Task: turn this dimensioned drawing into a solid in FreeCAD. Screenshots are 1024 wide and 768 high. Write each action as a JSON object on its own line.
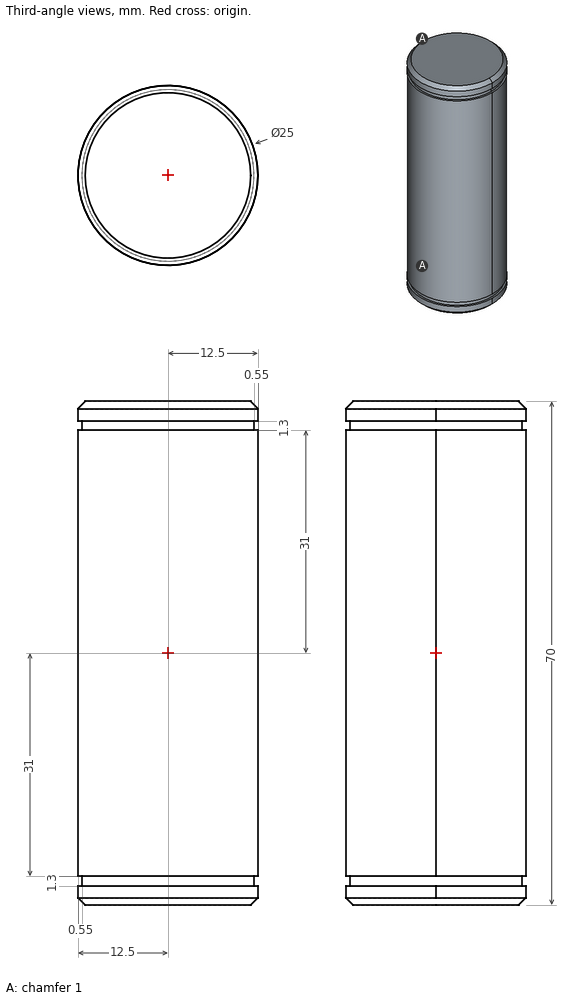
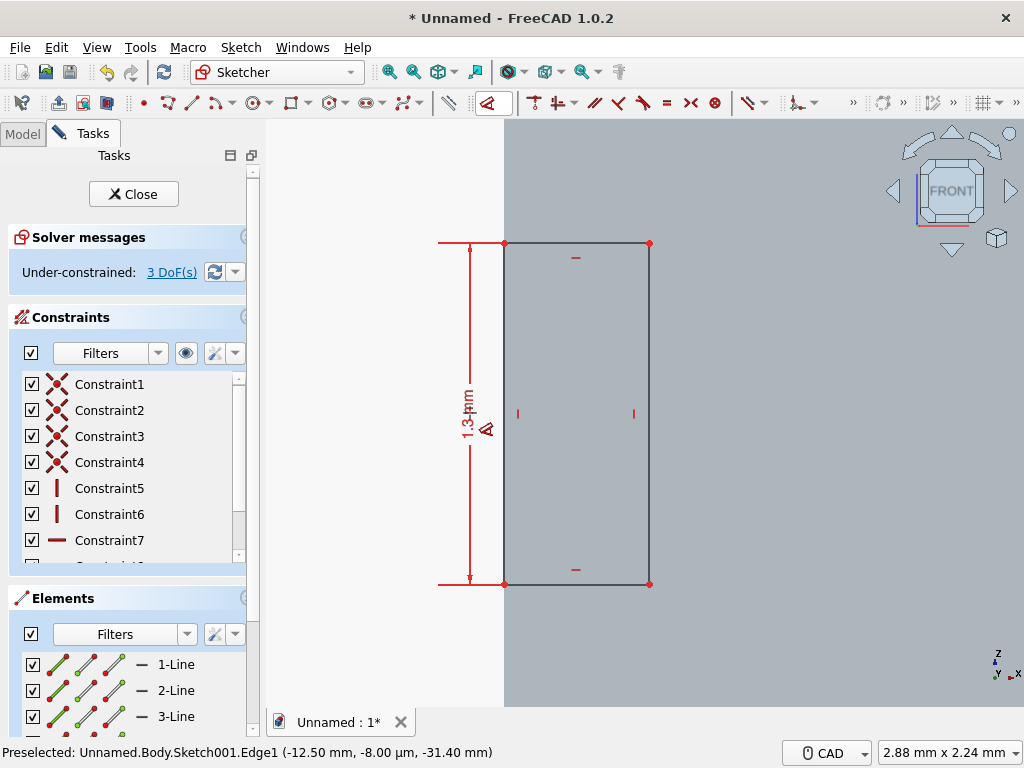
{"action": "left_click", "coordinate": [504, 243]}
{"action": "left_click", "coordinate": [470, 195]}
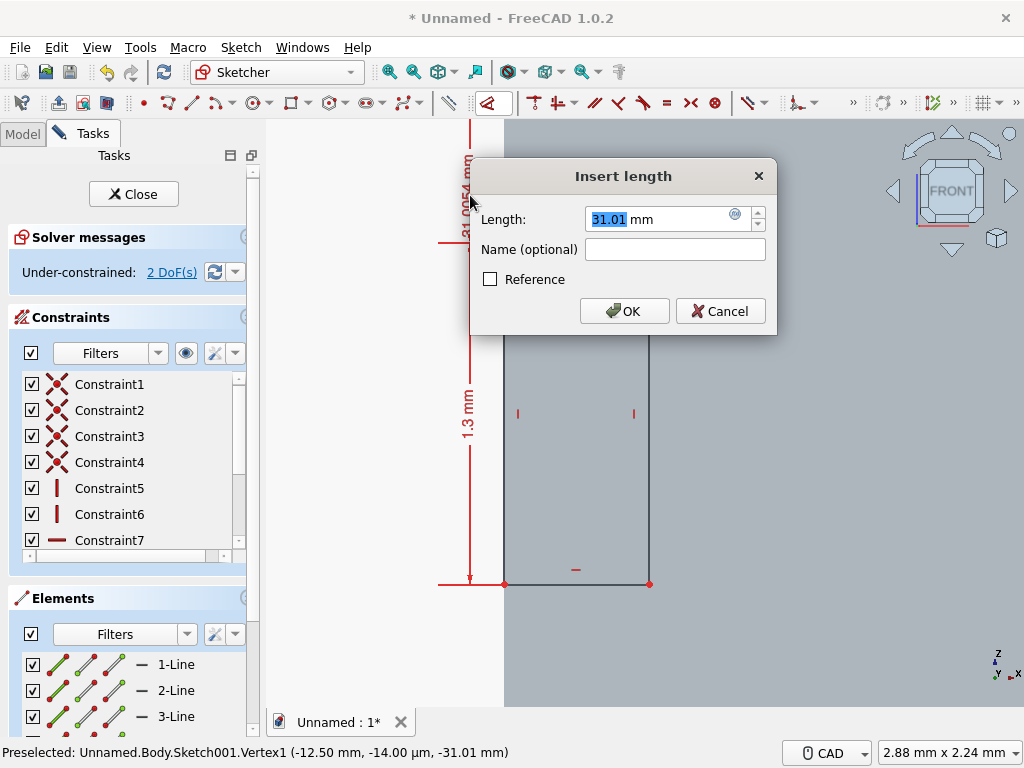
{"action": "type", "text": "31"}
{"action": "key", "text": "Return"}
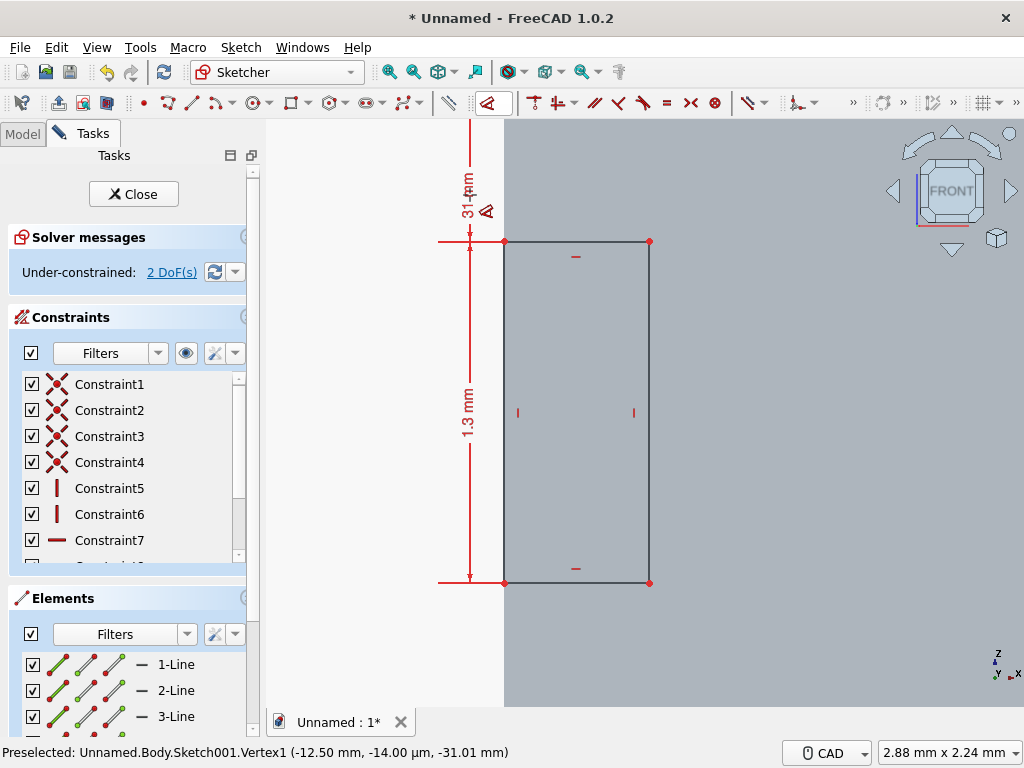
{"action": "left_click", "coordinate": [548, 583]}
{"action": "left_click", "coordinate": [577, 617]}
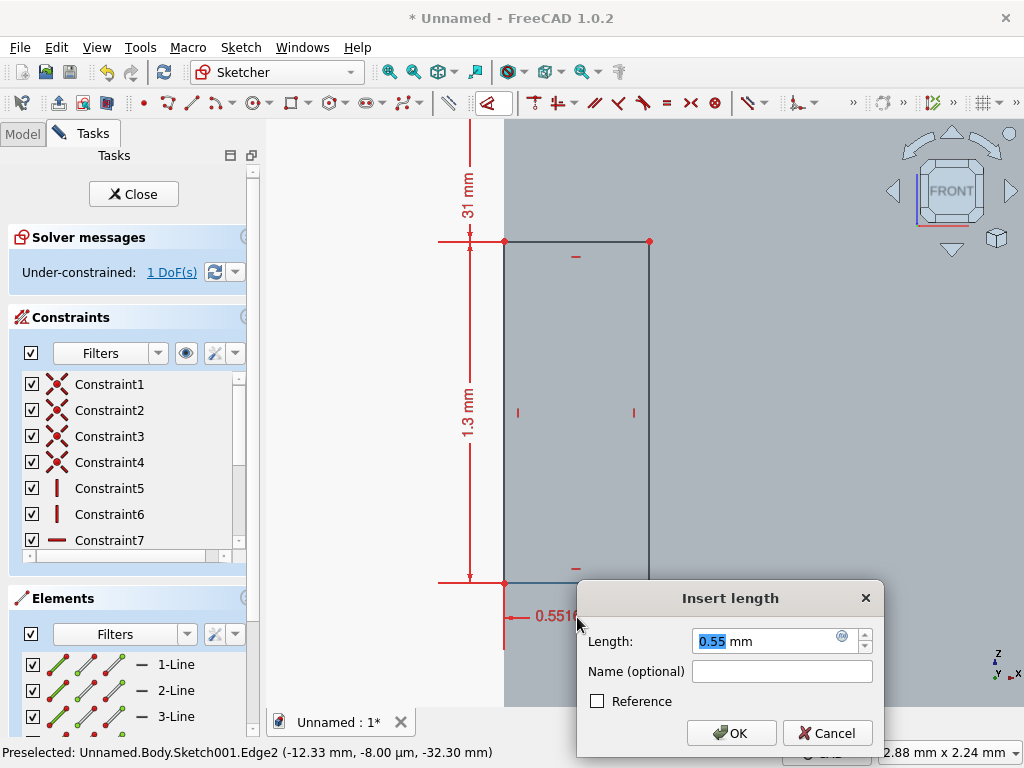
{"action": "type", "text": "0.55"}
{"action": "key", "text": "Return"}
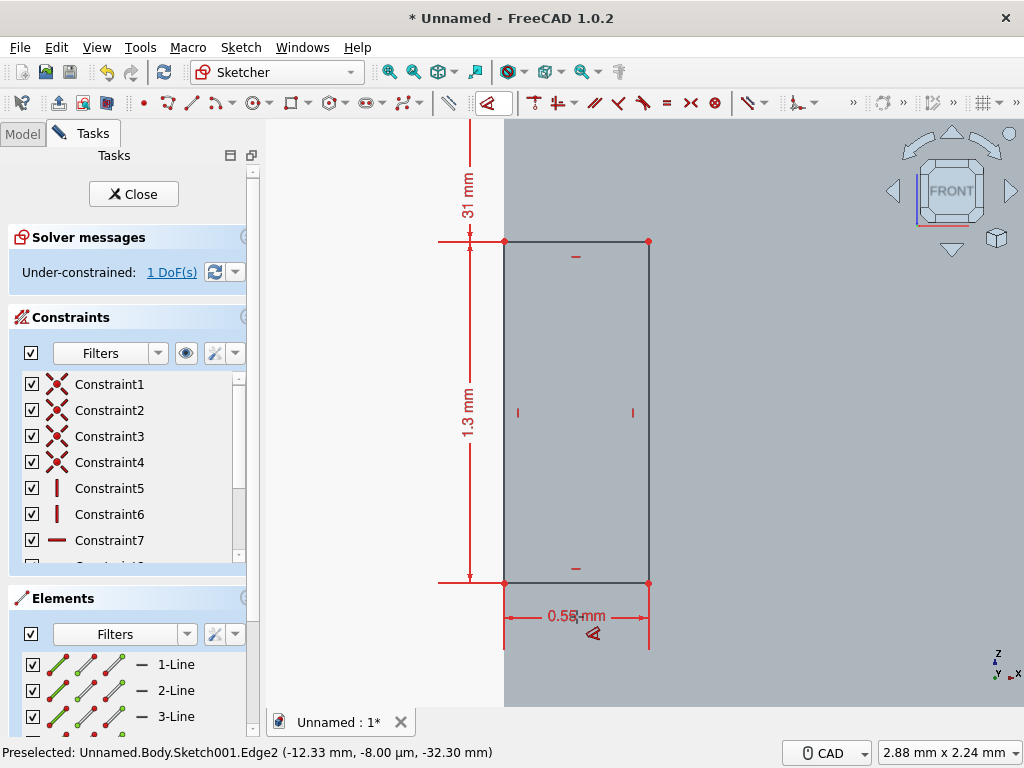
{"action": "left_click", "coordinate": [504, 242]}
{"action": "left_click", "coordinate": [682, 276]}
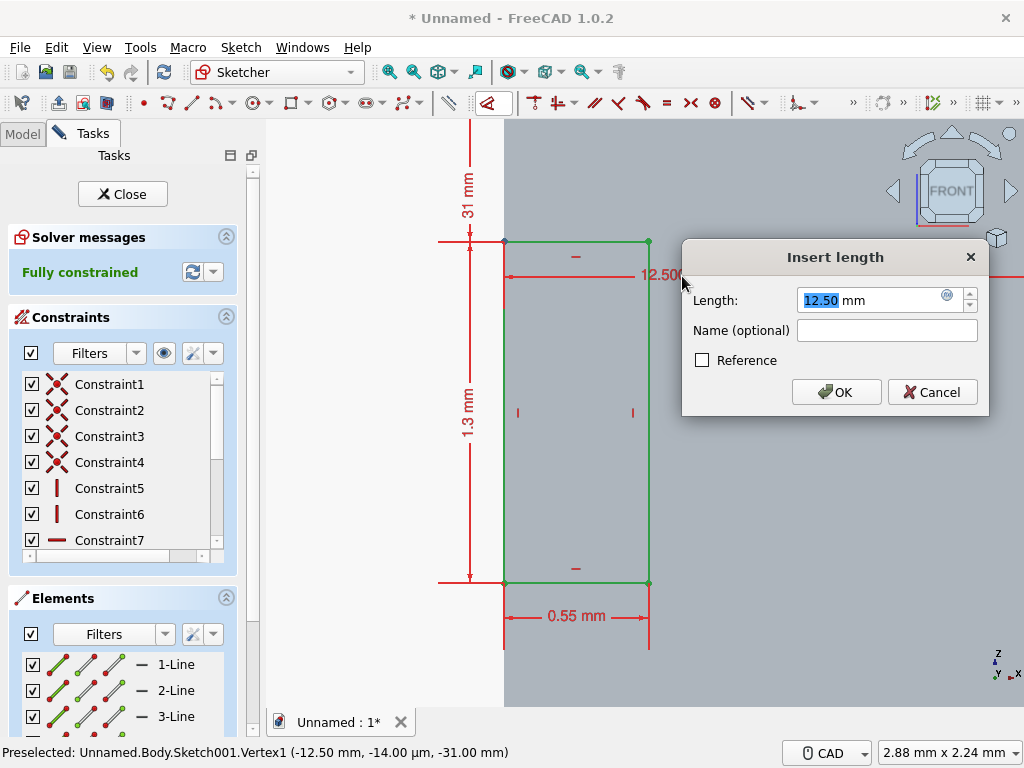
{"action": "type", "text": "12.5"}
{"action": "key", "text": "Return"}
{"action": "key", "text": "Escape"}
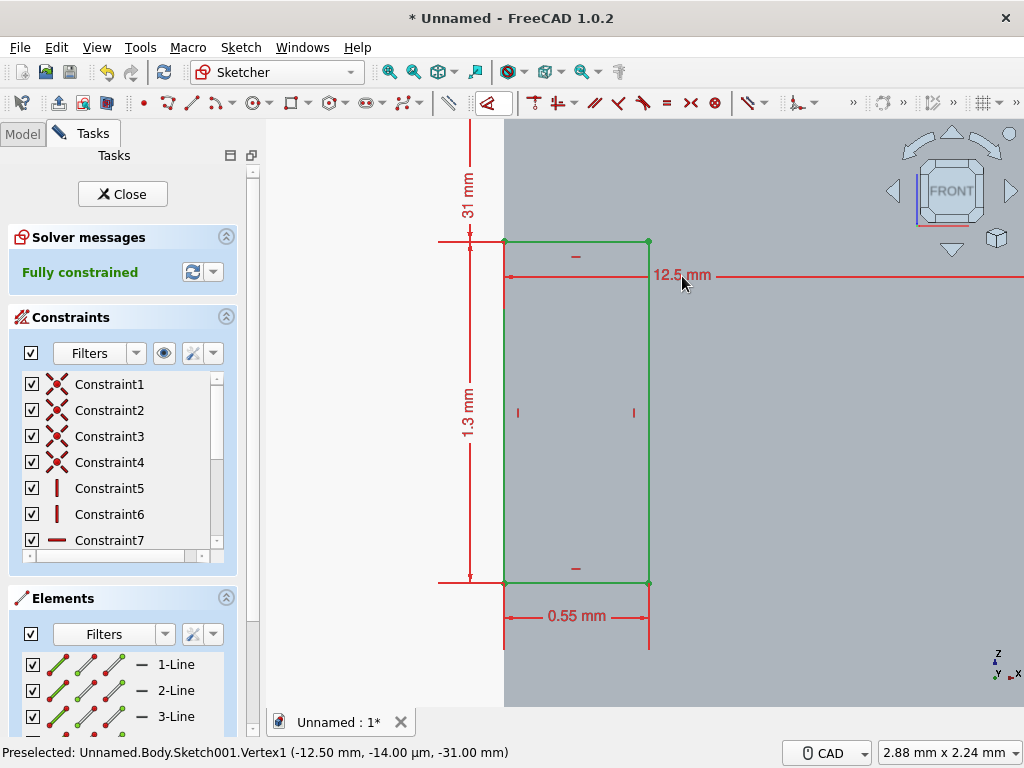
{"action": "left_click", "coordinate": [123, 194]}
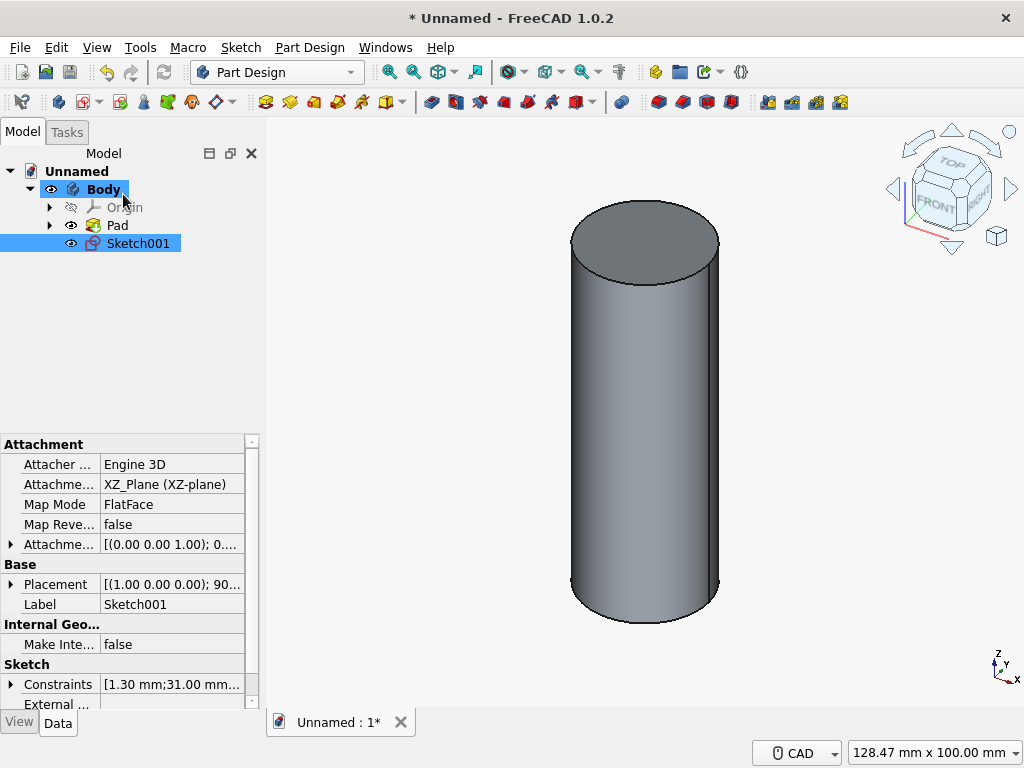
{"action": "left_click", "coordinate": [480, 102]}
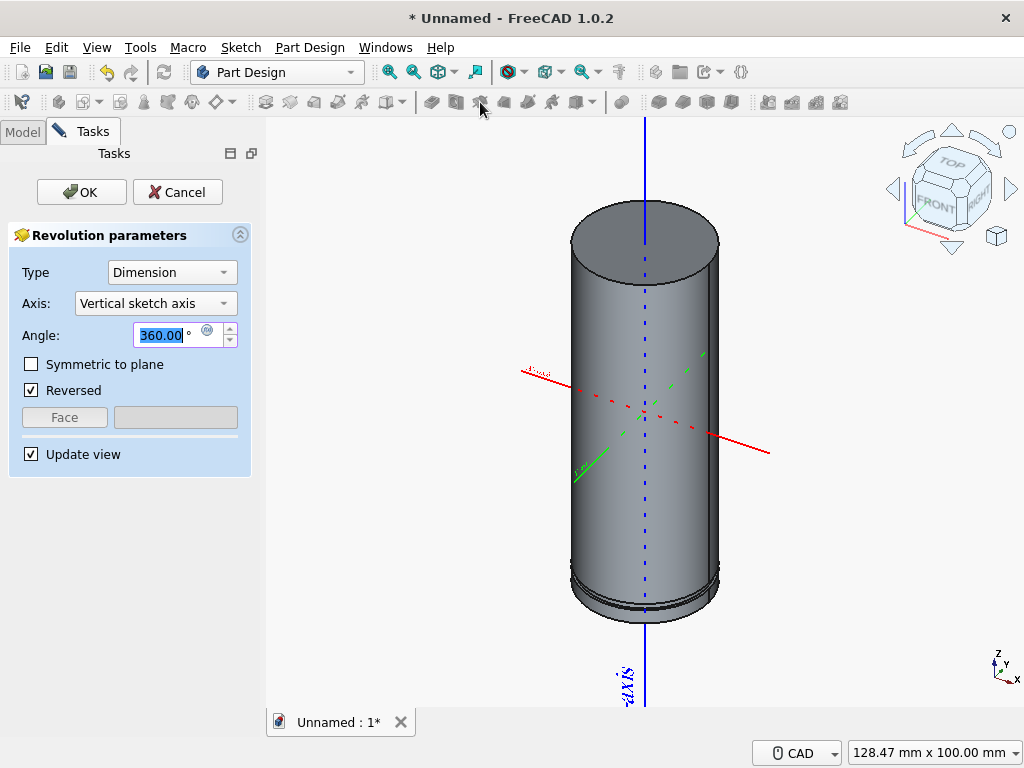
{"action": "left_click", "coordinate": [82, 192]}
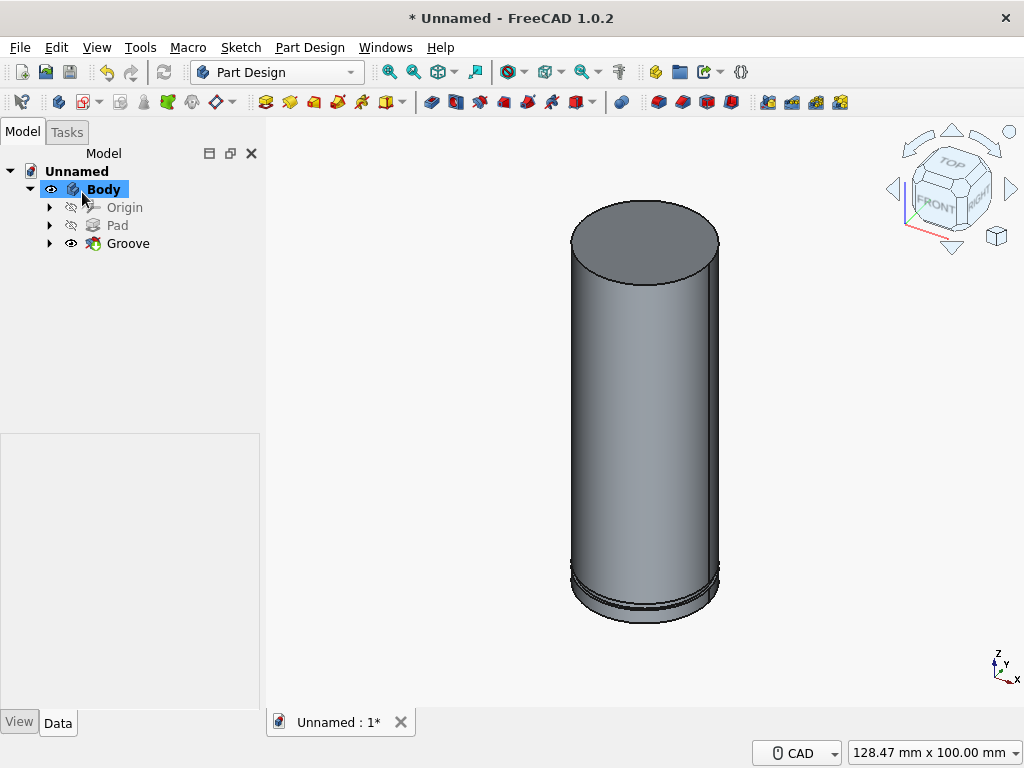
{"action": "left_click", "coordinate": [84, 102]}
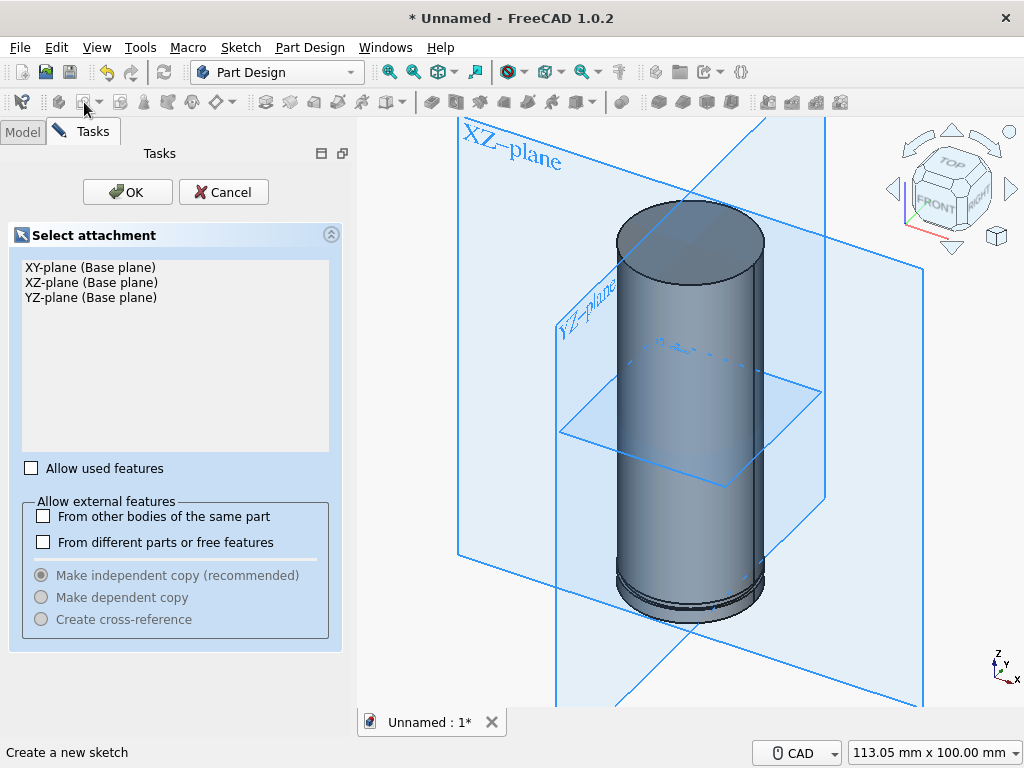
{"action": "left_click", "coordinate": [82, 282]}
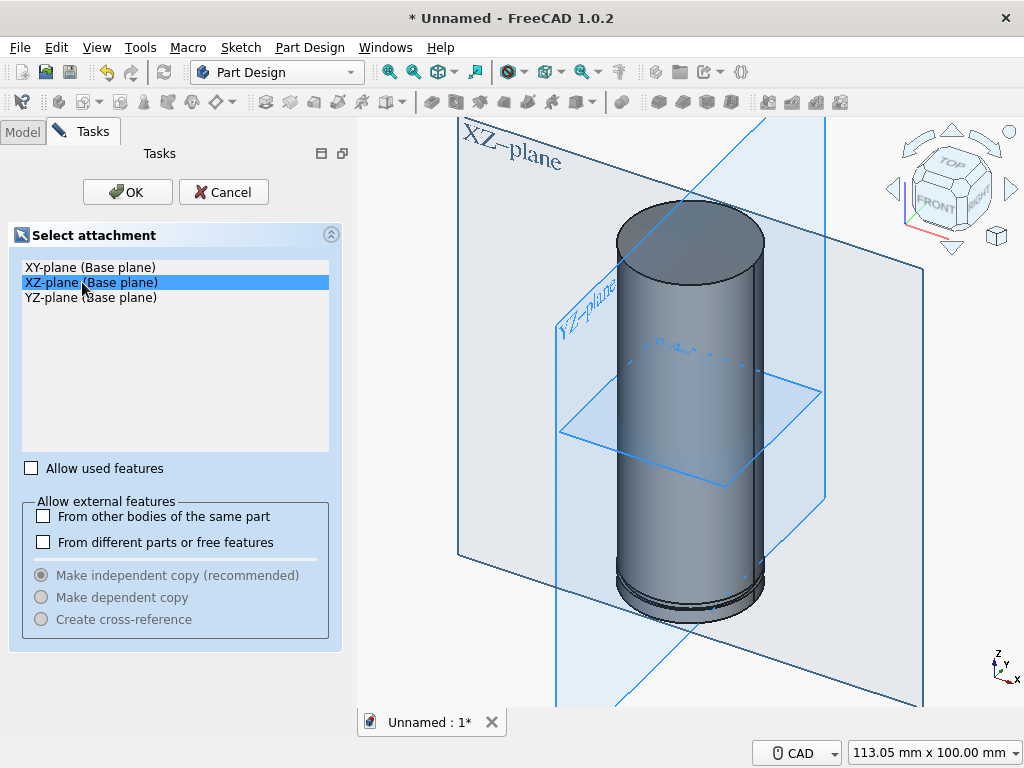
{"action": "left_click", "coordinate": [128, 192]}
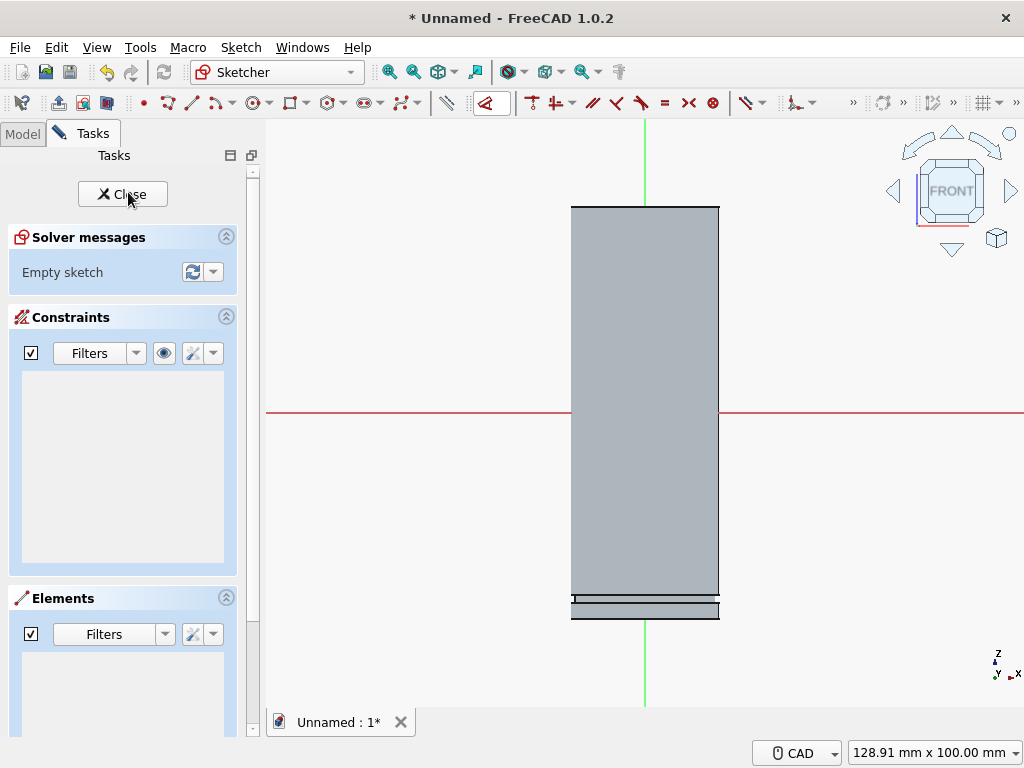
{"action": "key", "text": "q s"}